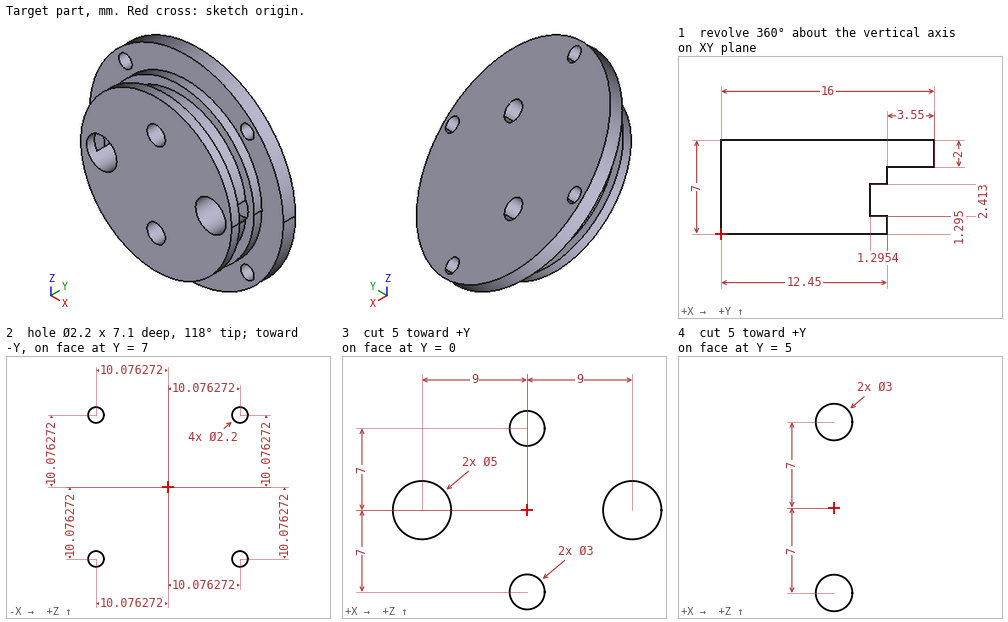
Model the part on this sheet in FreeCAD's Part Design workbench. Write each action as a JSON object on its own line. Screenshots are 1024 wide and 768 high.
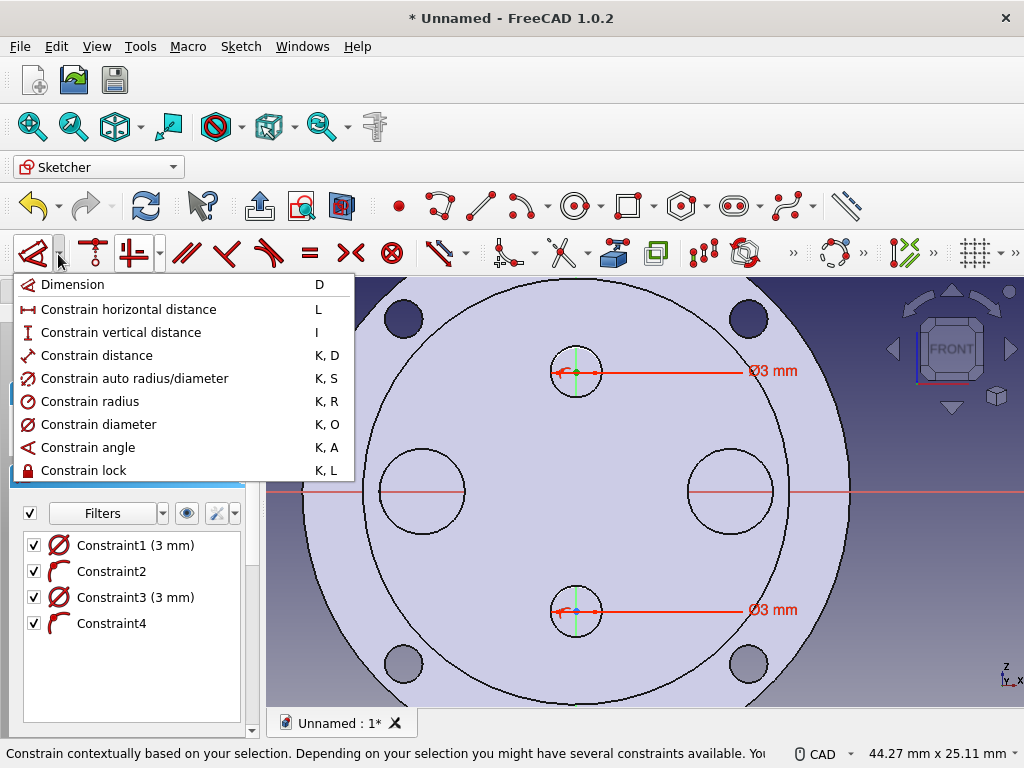
{"action": "left_click", "coordinate": [184, 332]}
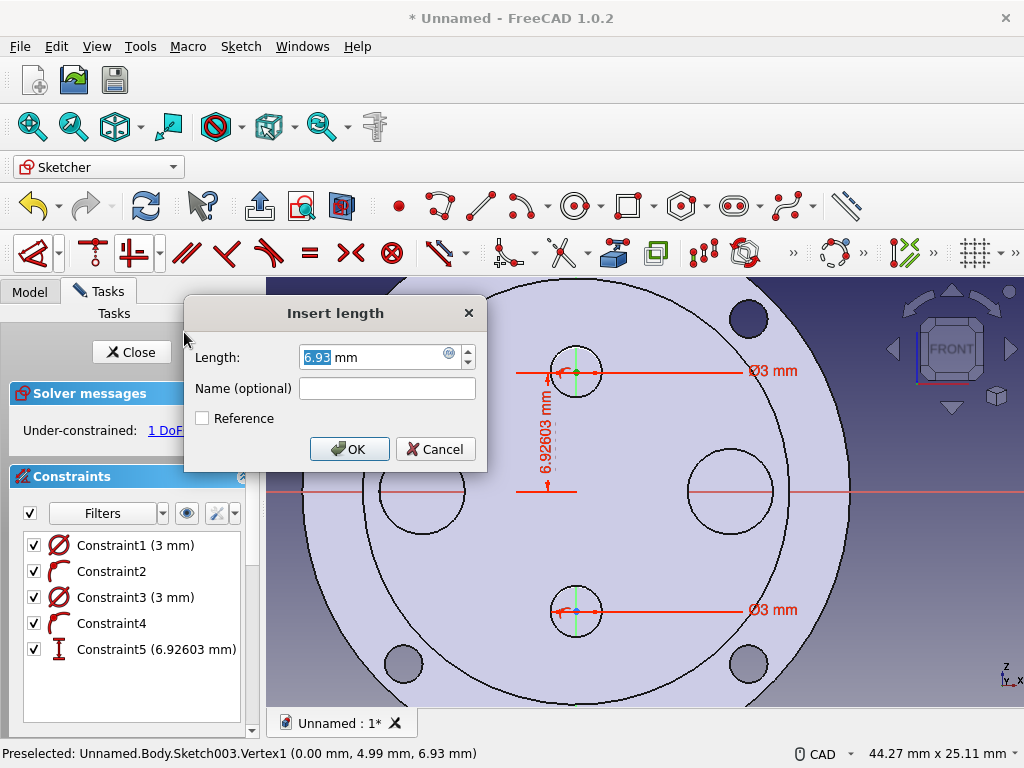
{"action": "type", "text": "7"}
{"action": "key", "text": "Return"}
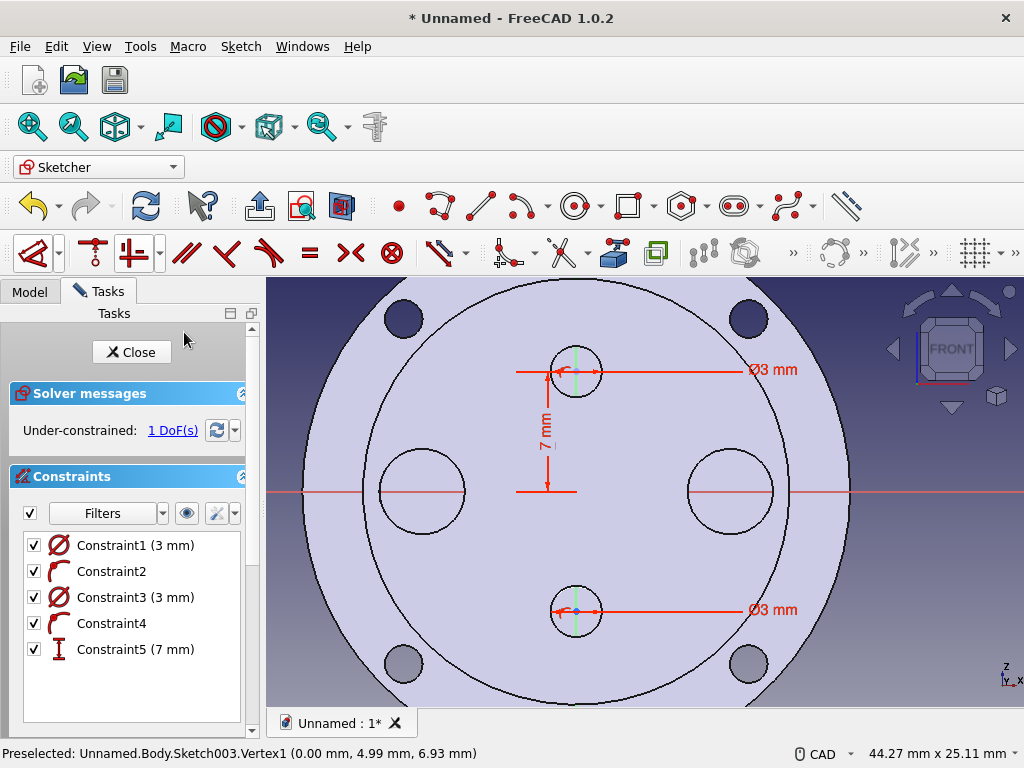
{"action": "left_click", "coordinate": [576, 612]}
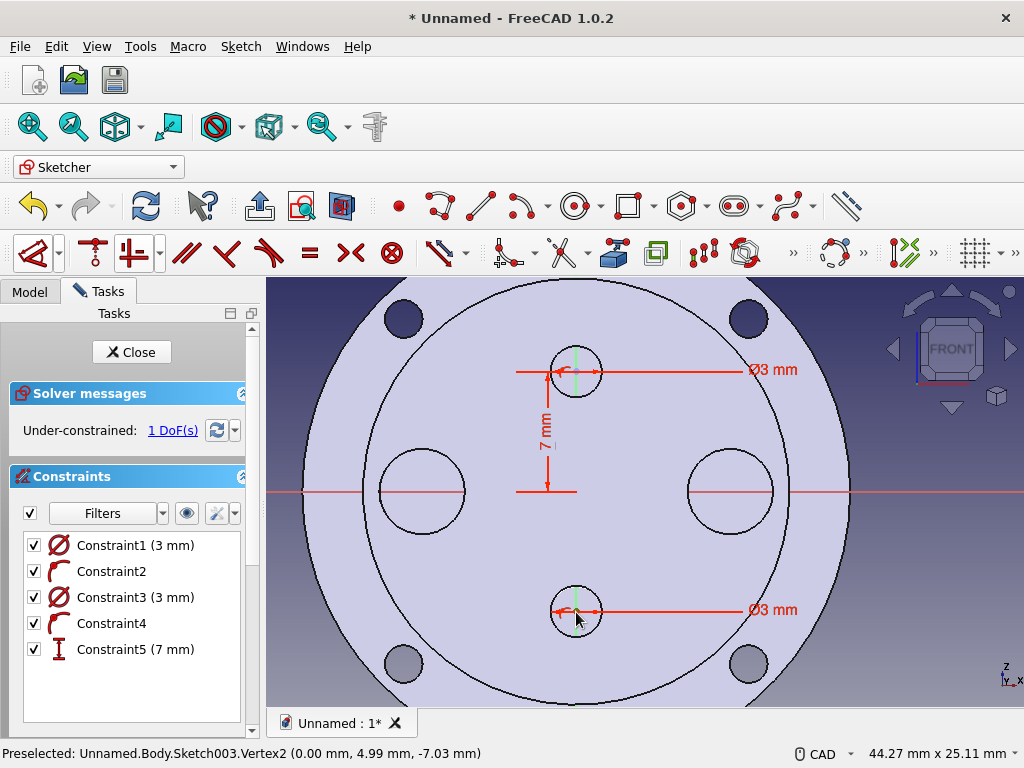
{"action": "left_click", "coordinate": [58, 254]}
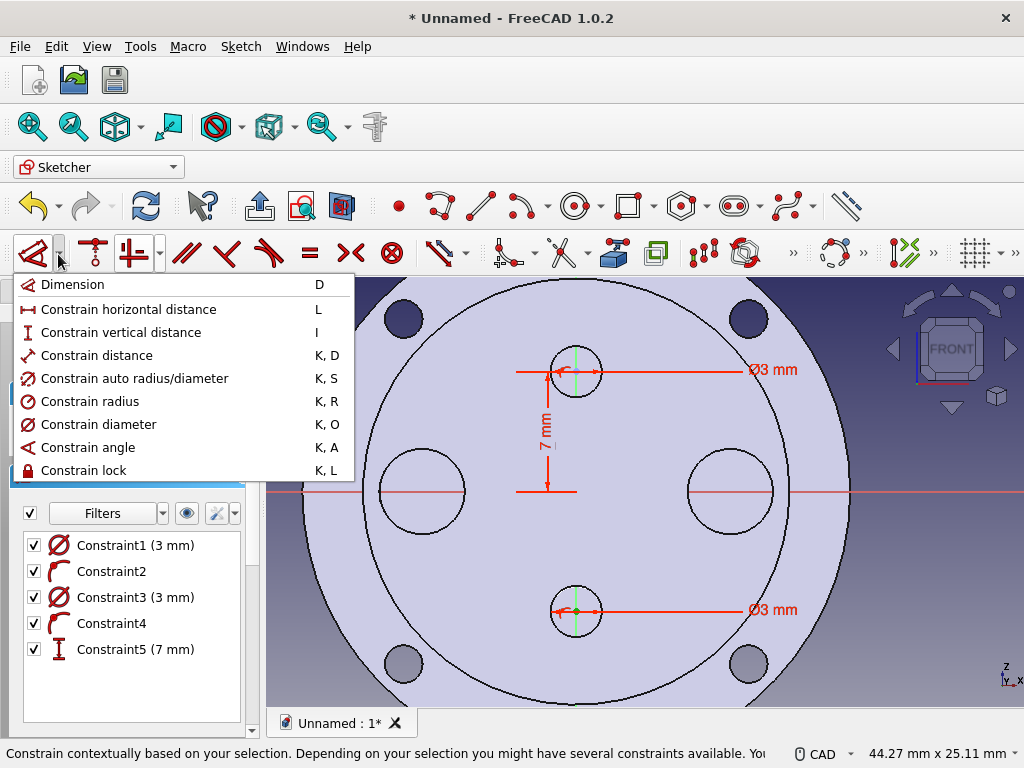
{"action": "left_click", "coordinate": [184, 332]}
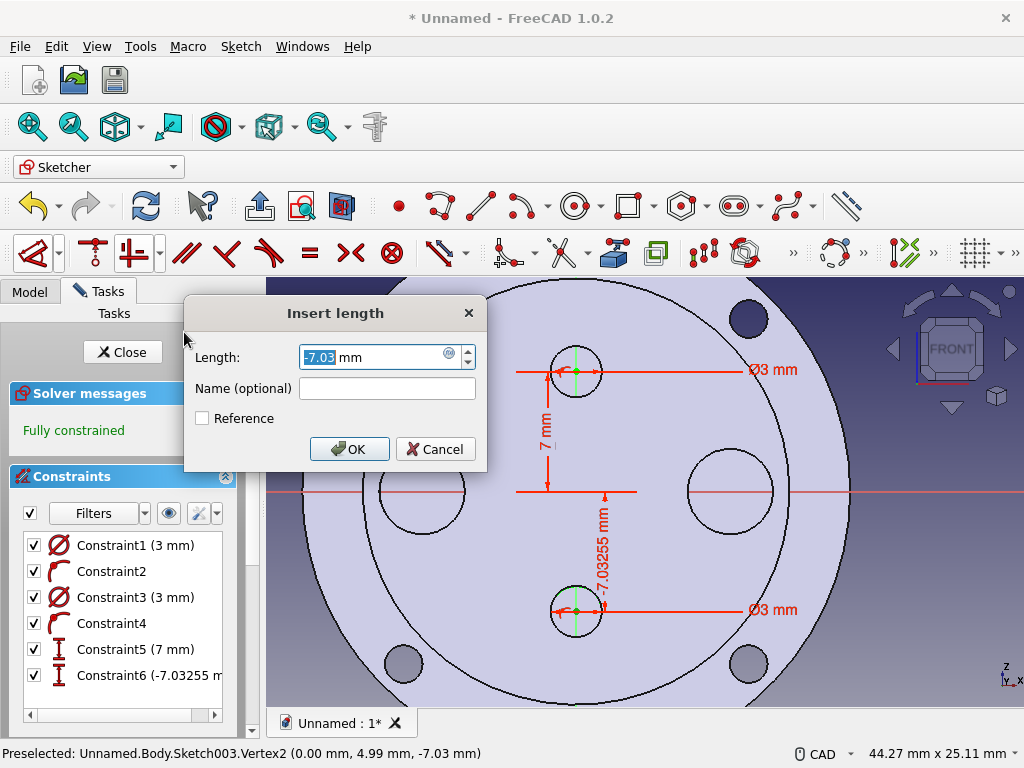
{"action": "type", "text": "-7"}
{"action": "key", "text": "Return"}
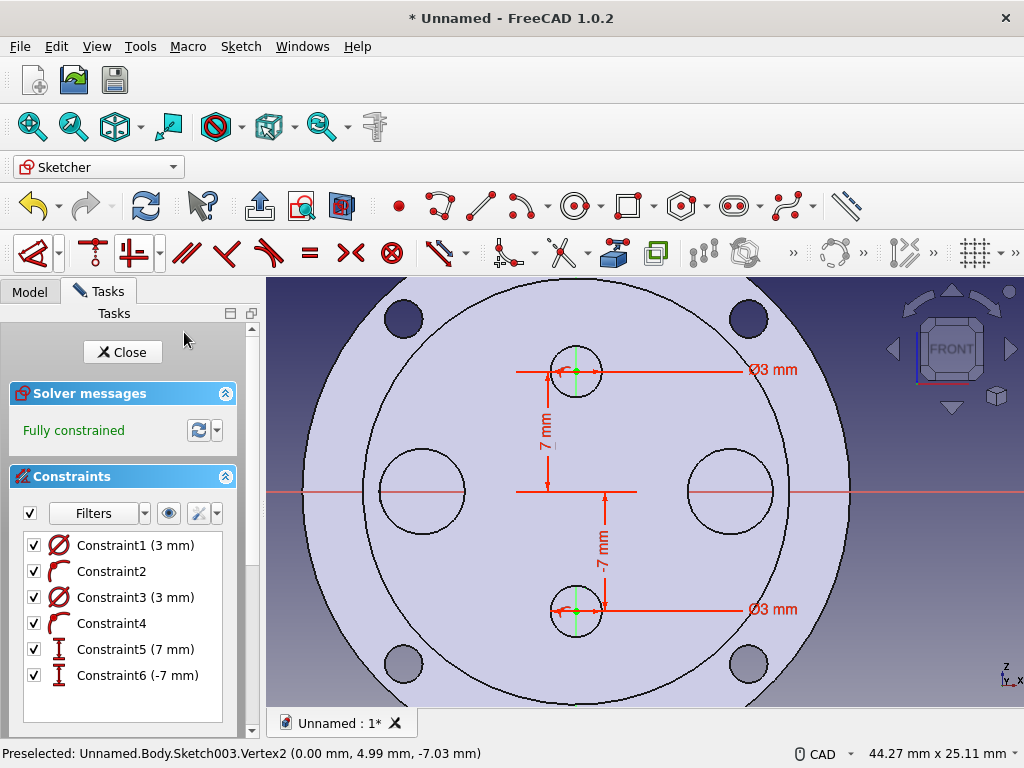
{"action": "left_click", "coordinate": [123, 352]}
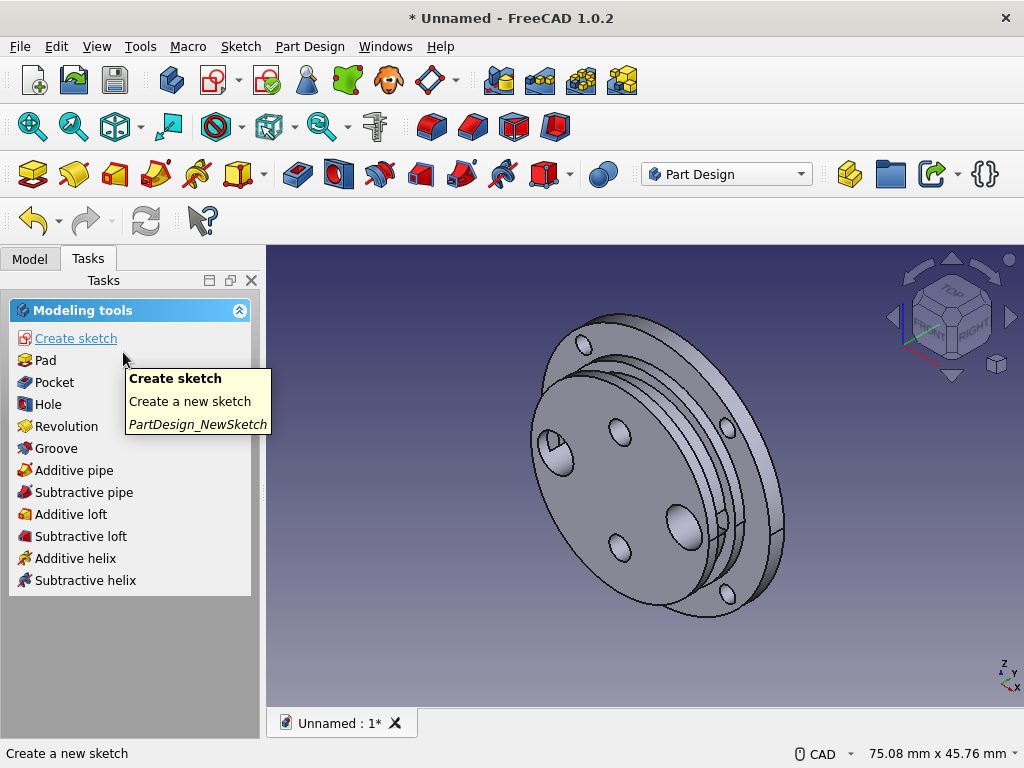
{"action": "left_click", "coordinate": [298, 174]}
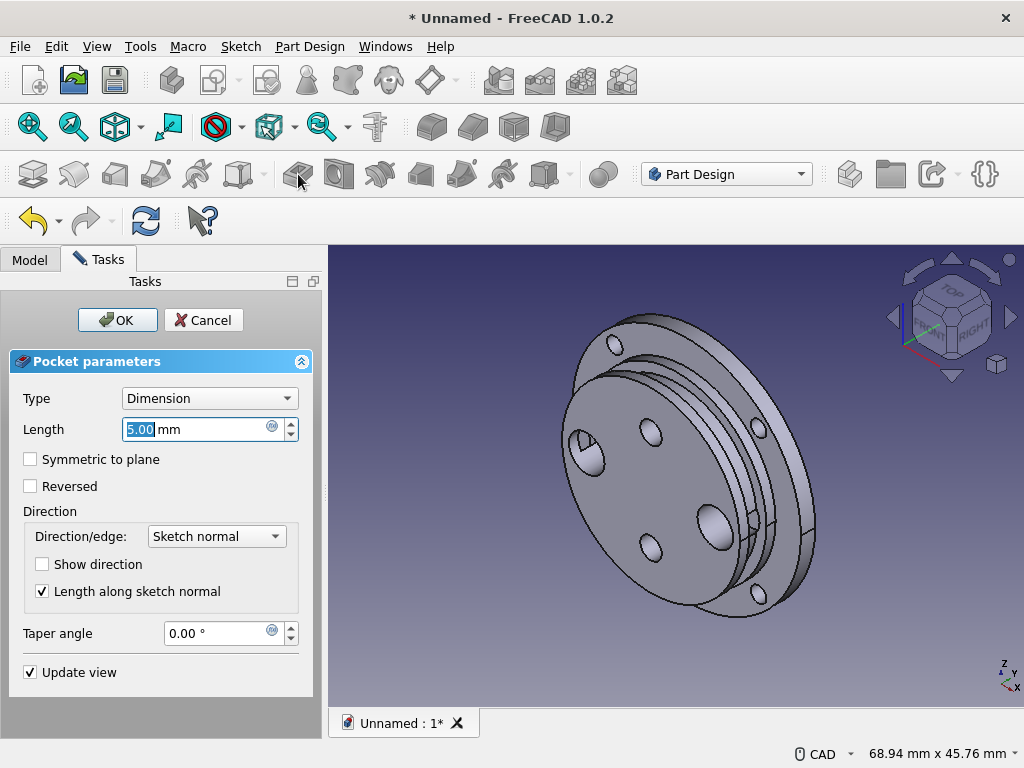
{"action": "type", "text": "5"}
{"action": "key", "text": "Tab"}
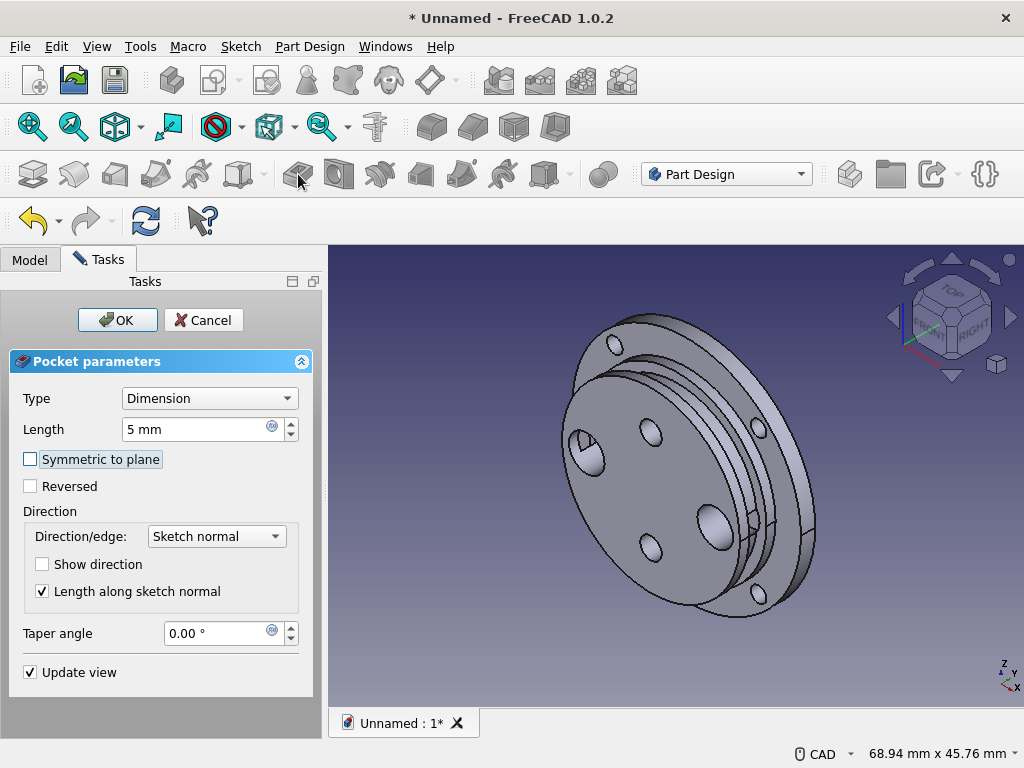
{"action": "left_click", "coordinate": [118, 320]}